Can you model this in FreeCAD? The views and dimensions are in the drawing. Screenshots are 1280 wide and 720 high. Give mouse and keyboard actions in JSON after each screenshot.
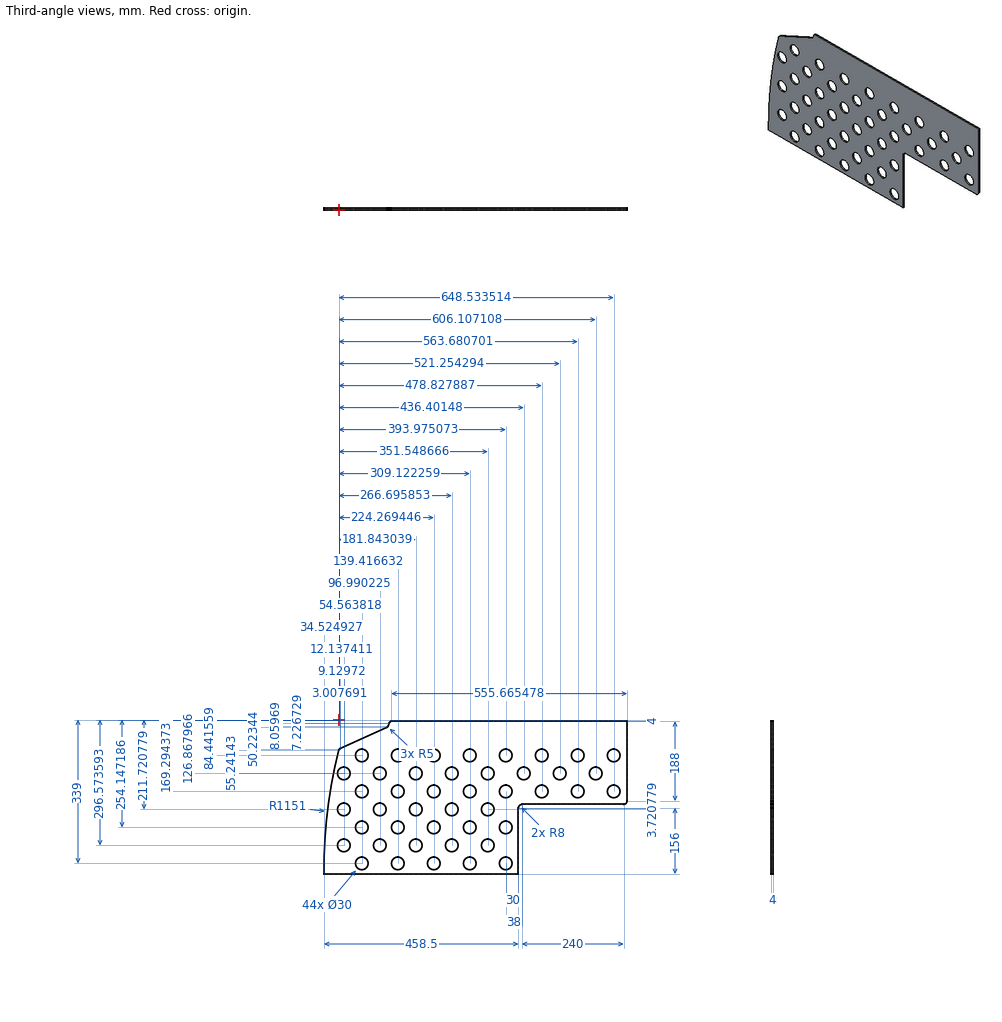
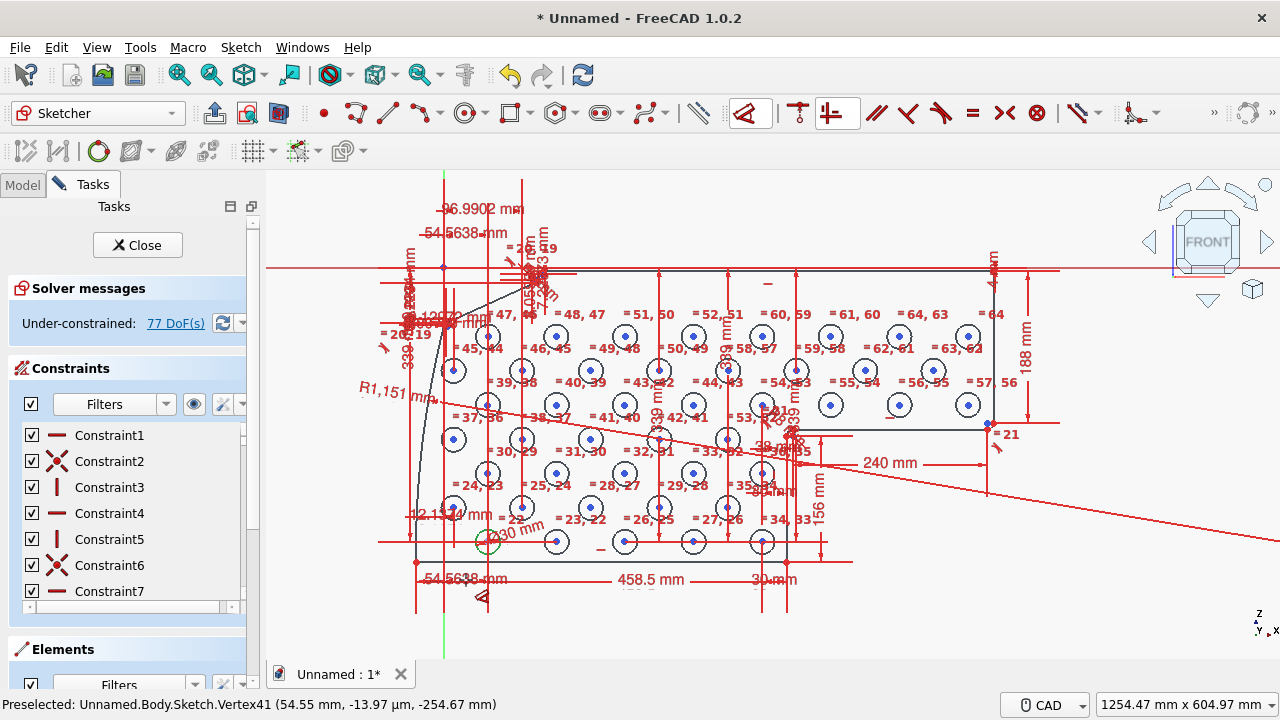
{"action": "scroll", "coordinate": [454, 440], "scroll_direction": "up", "scroll_amount": 7}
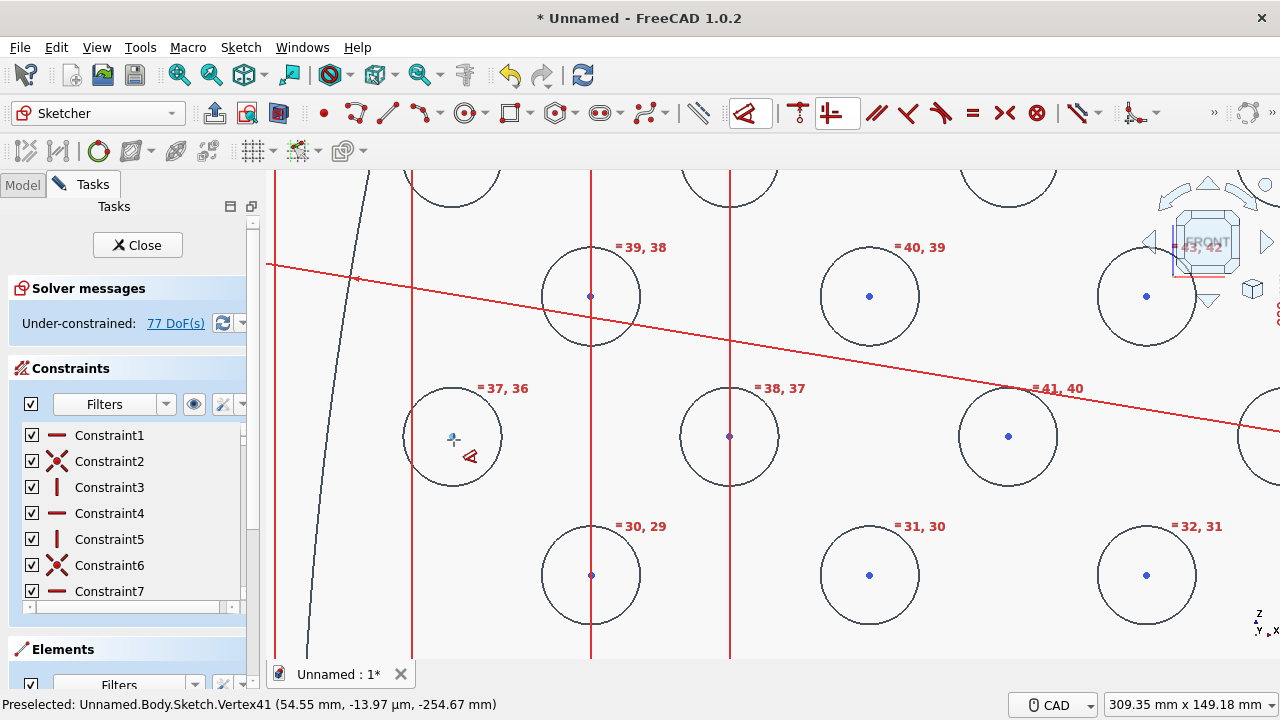
{"action": "left_click", "coordinate": [453, 437]}
{"action": "left_click", "coordinate": [442, 471]}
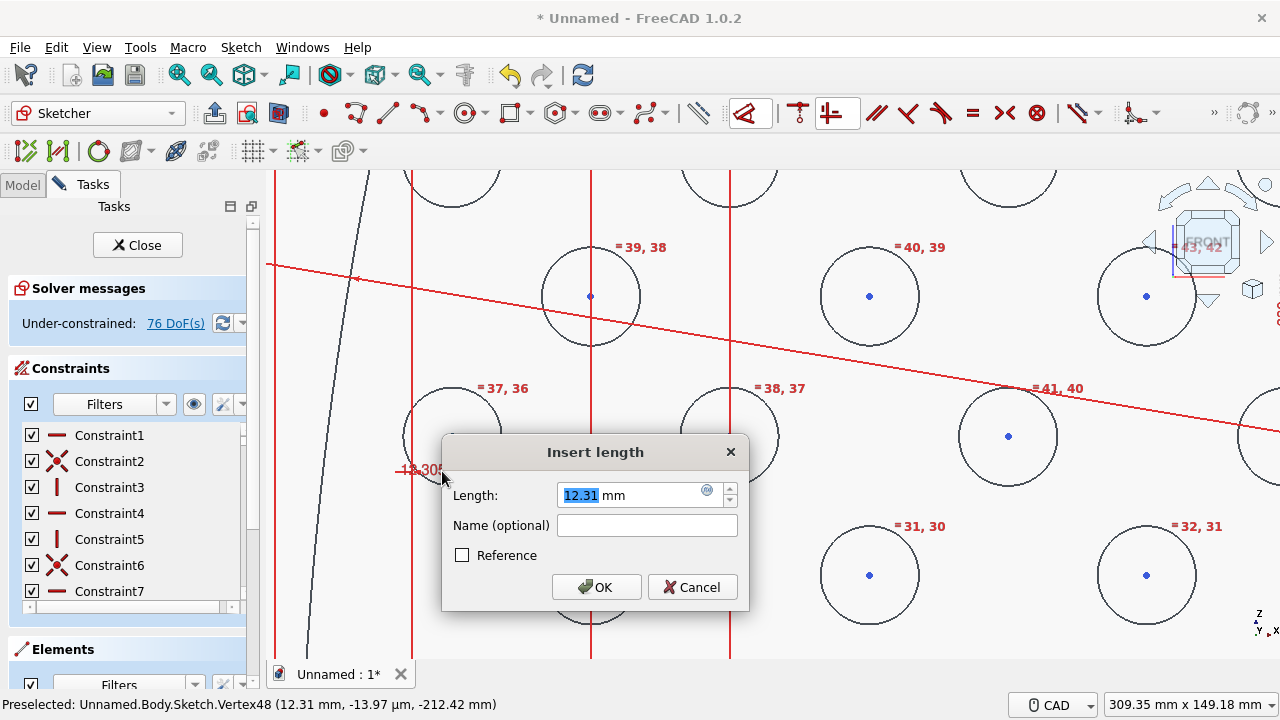
{"action": "type", "text": "12.137411"}
{"action": "key", "text": "Return"}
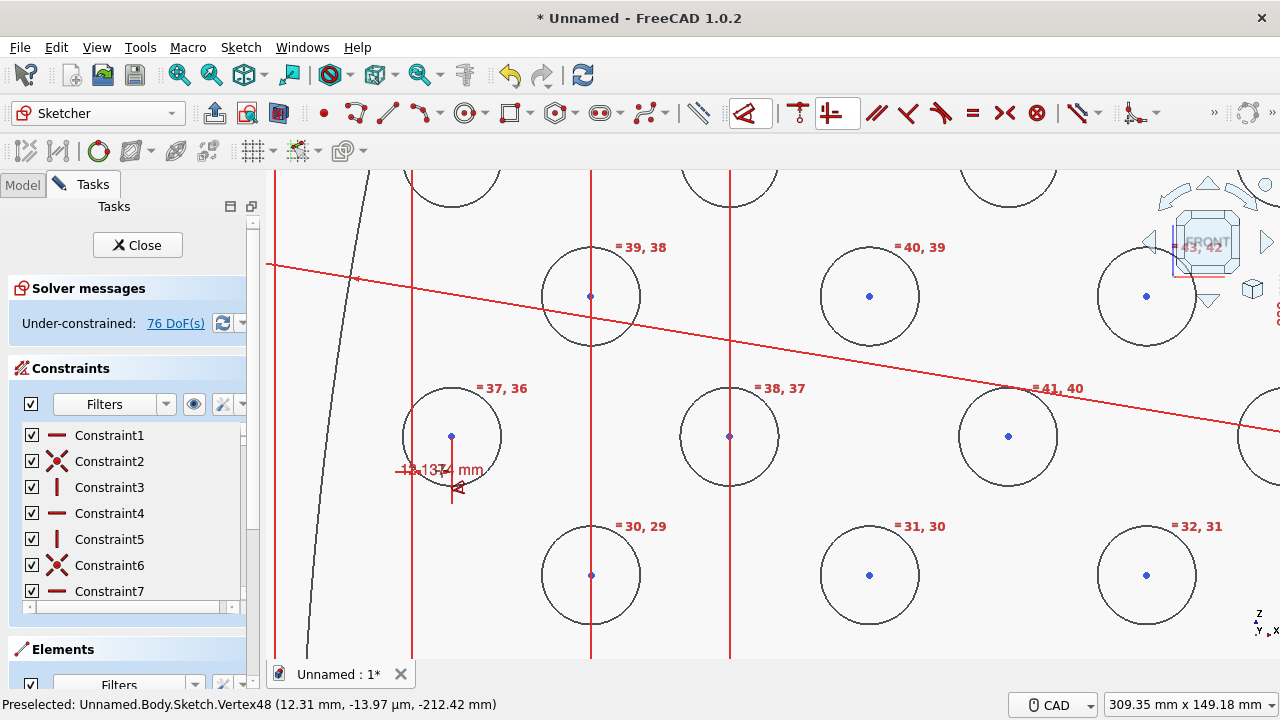
{"action": "scroll", "coordinate": [454, 440], "scroll_direction": "down", "scroll_amount": 7}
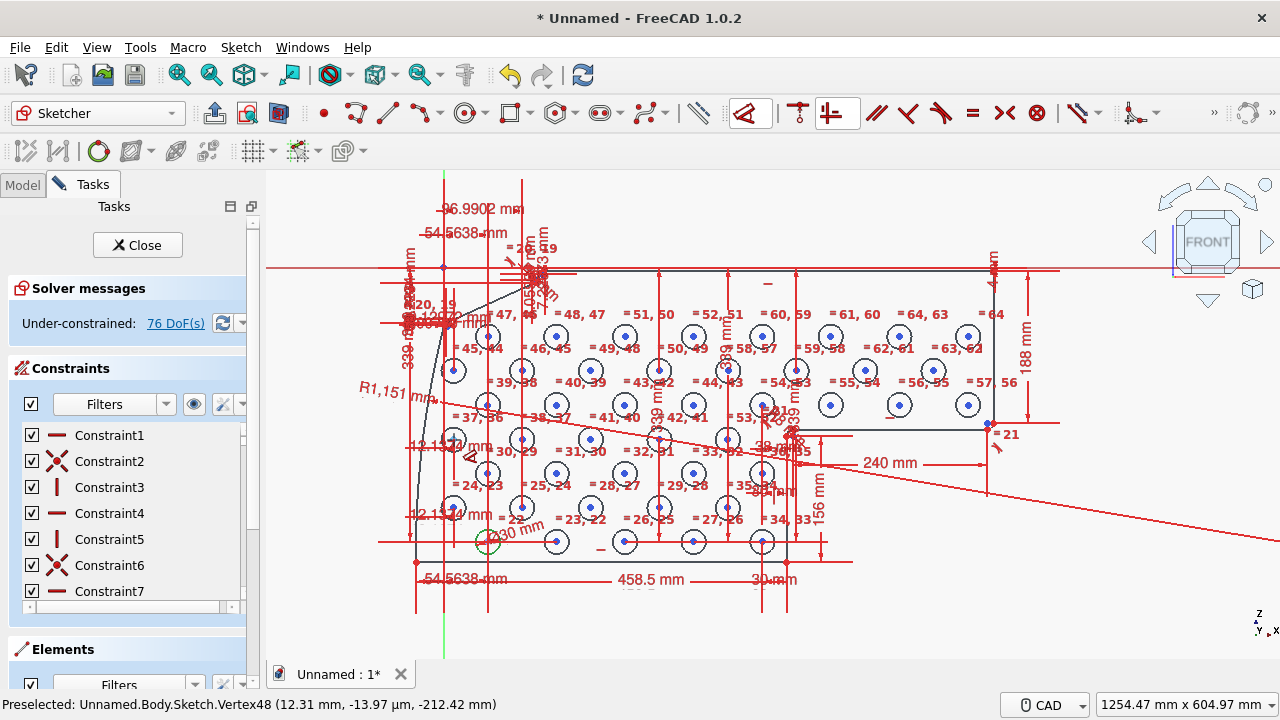
{"action": "left_click", "coordinate": [522, 440]}
{"action": "left_click", "coordinate": [483, 620]}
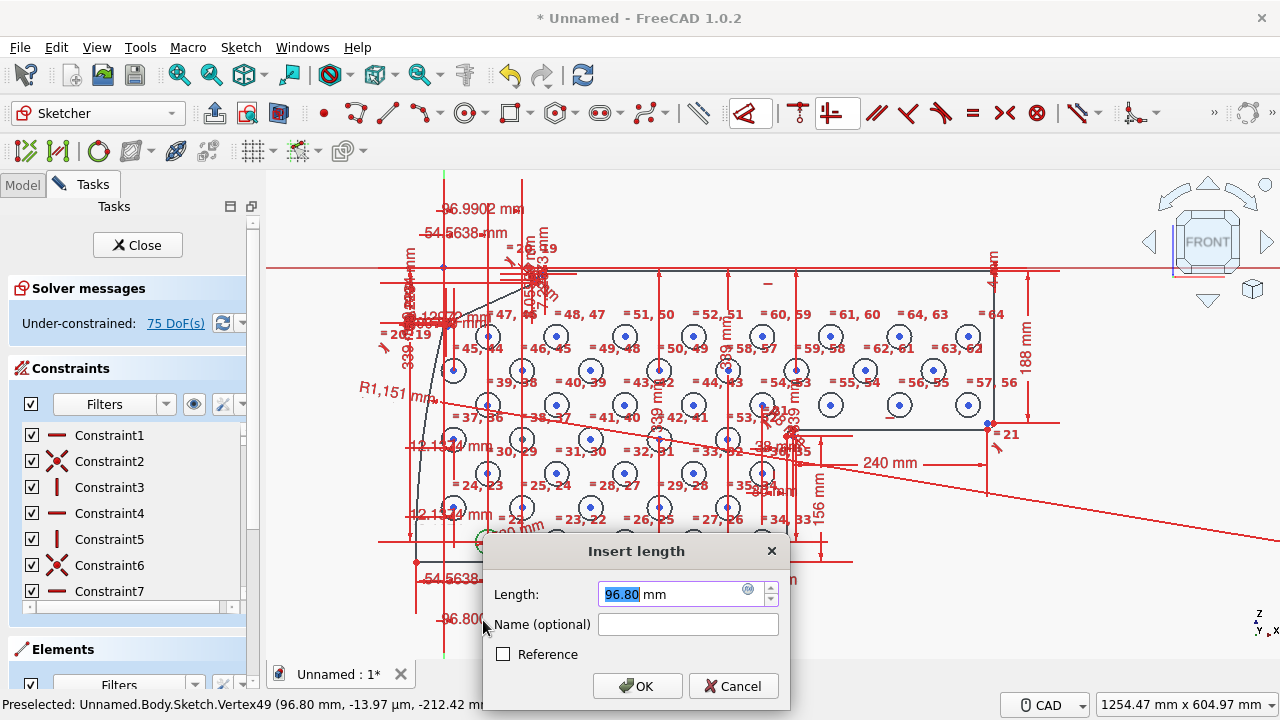
{"action": "type", "text": "96.990225"}
{"action": "key", "text": "Return"}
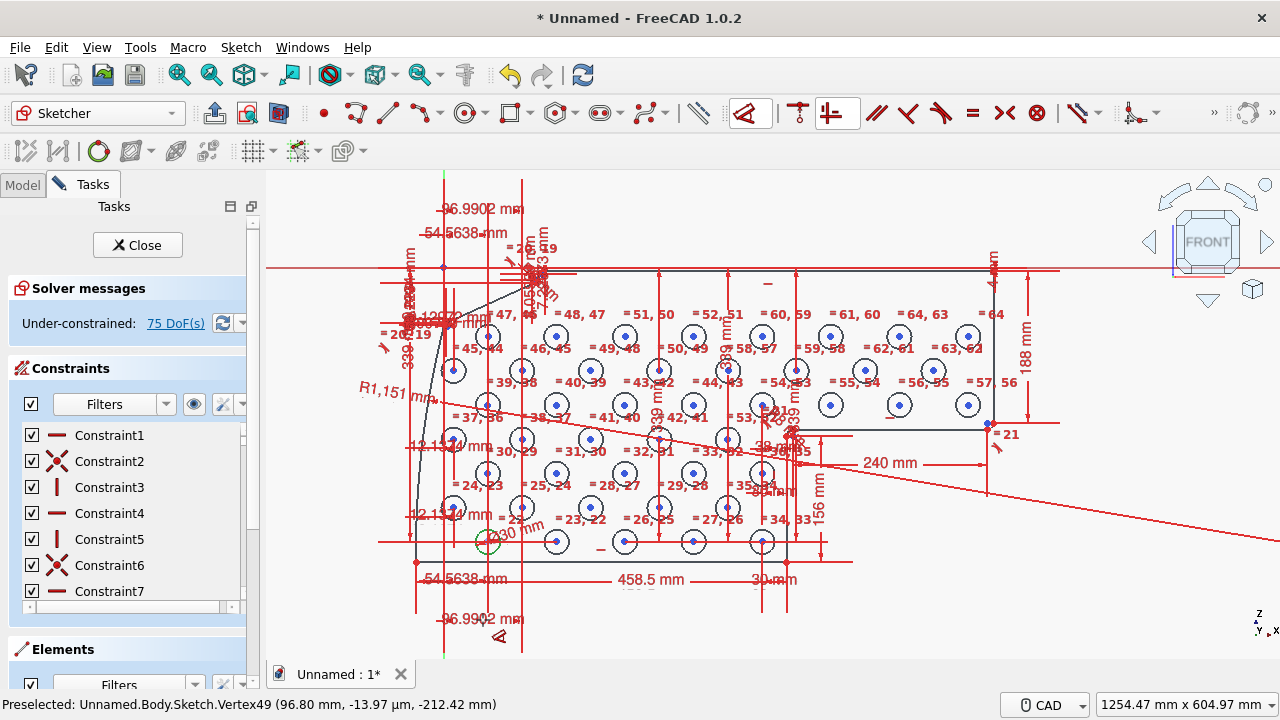
{"action": "left_click", "coordinate": [488, 405]}
{"action": "left_click", "coordinate": [466, 463]}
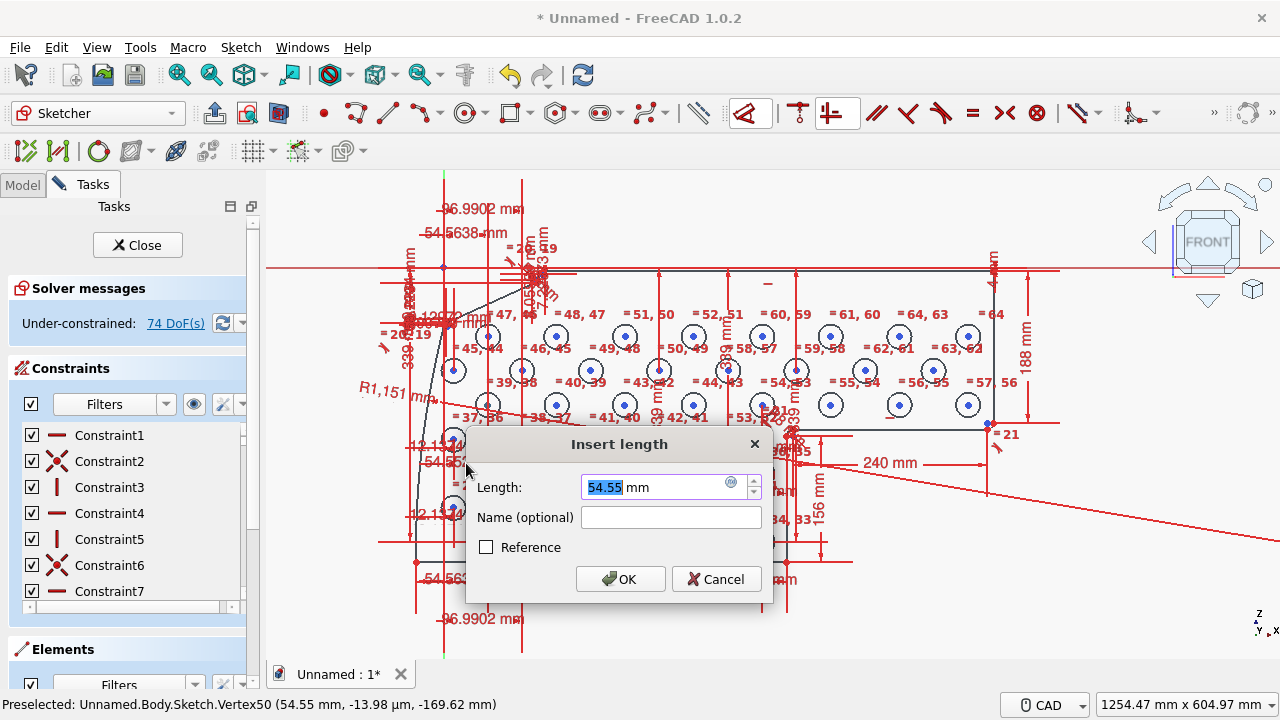
{"action": "type", "text": "54.563818"}
{"action": "key", "text": "Return"}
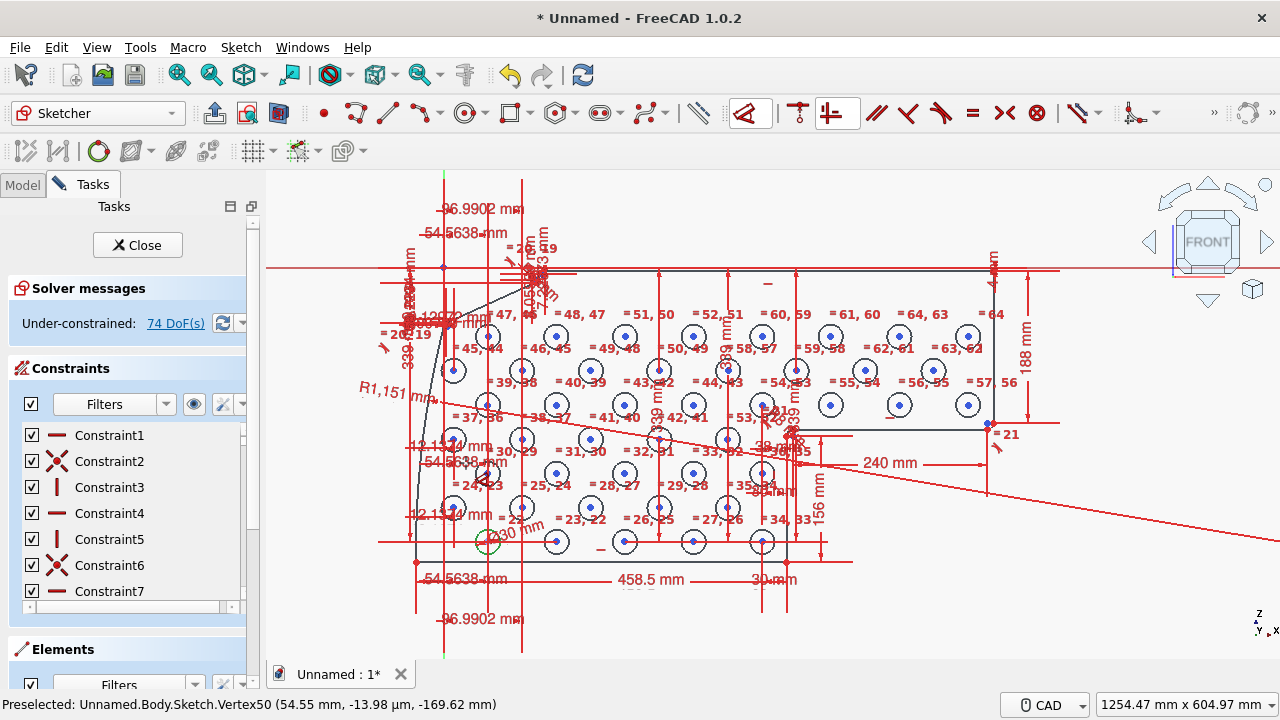
{"action": "left_click", "coordinate": [522, 371]}
{"action": "left_click", "coordinate": [501, 234]}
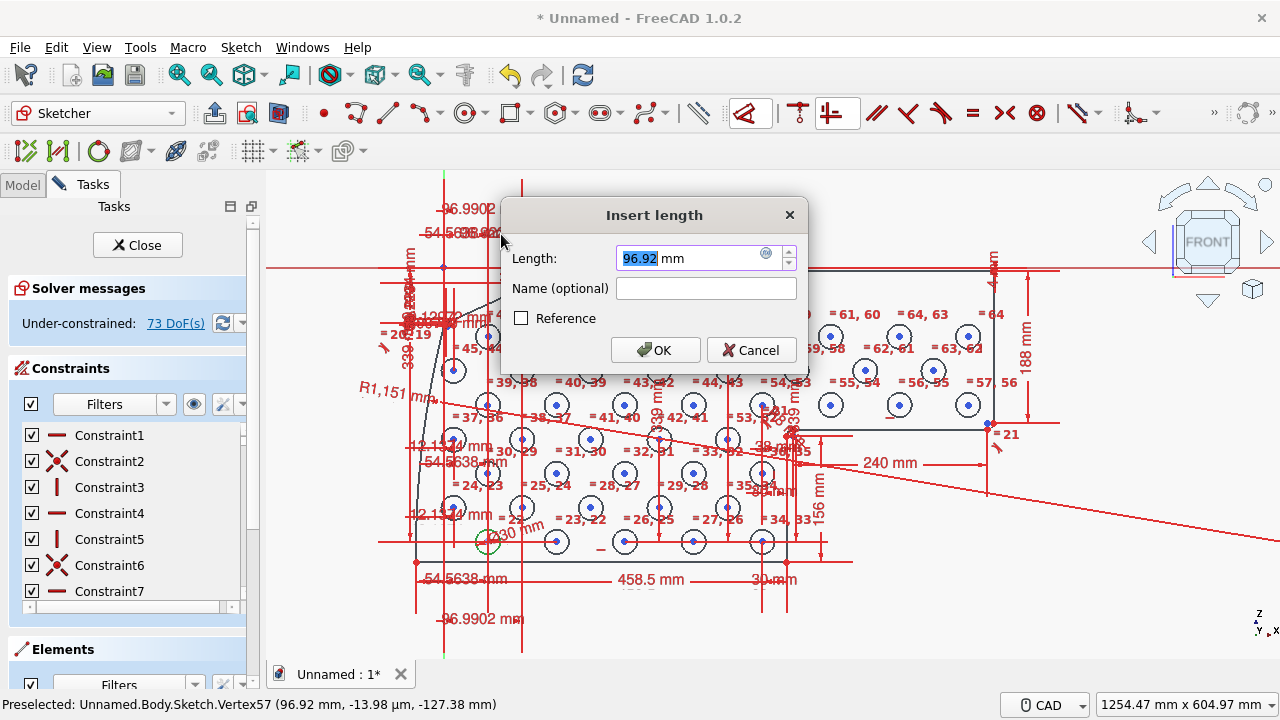
{"action": "type", "text": "96.990225"}
{"action": "key", "text": "Return"}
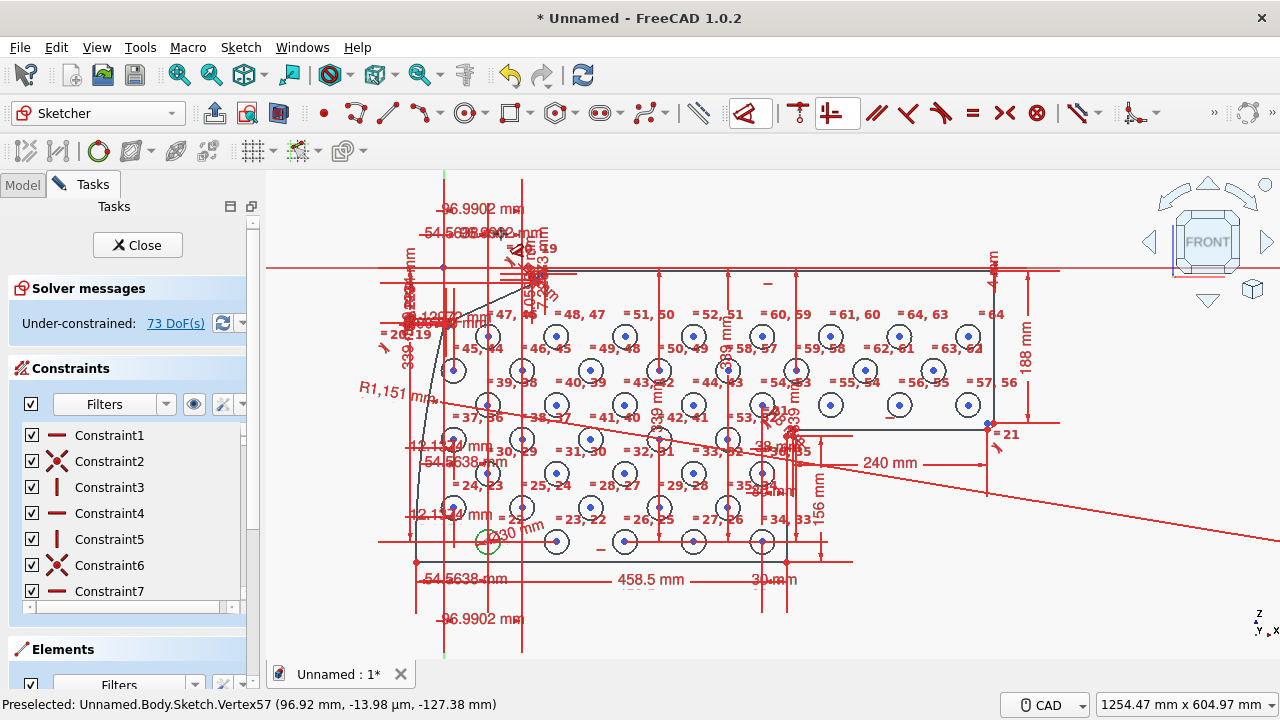
{"action": "left_click", "coordinate": [488, 337]}
{"action": "left_click", "coordinate": [481, 371]}